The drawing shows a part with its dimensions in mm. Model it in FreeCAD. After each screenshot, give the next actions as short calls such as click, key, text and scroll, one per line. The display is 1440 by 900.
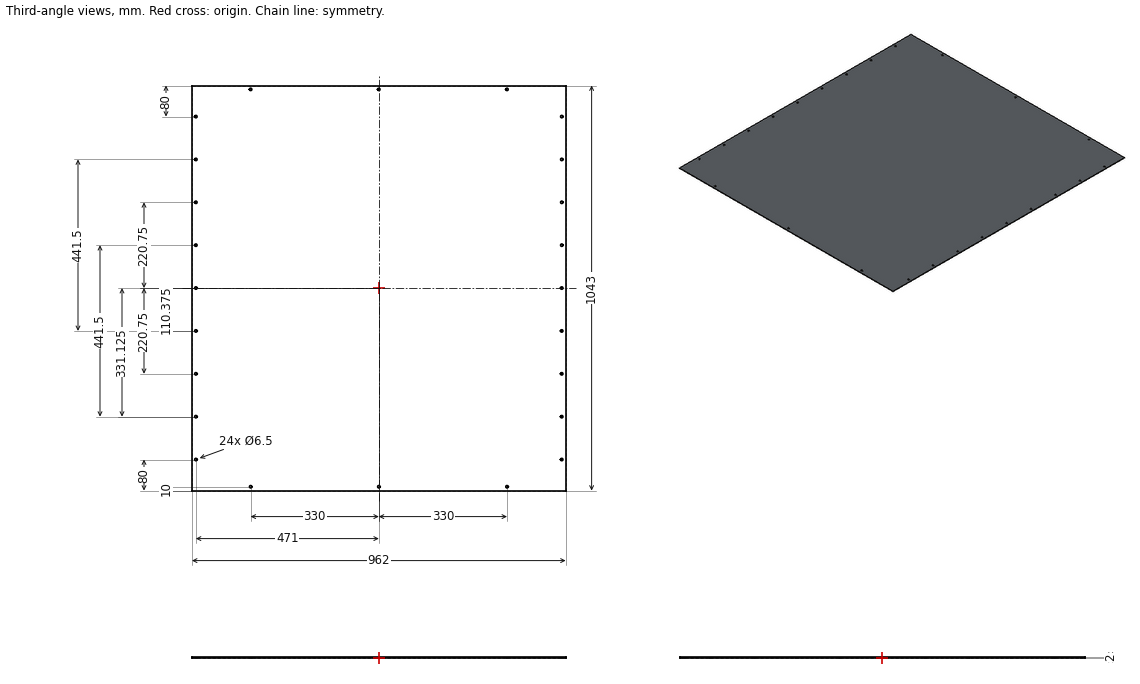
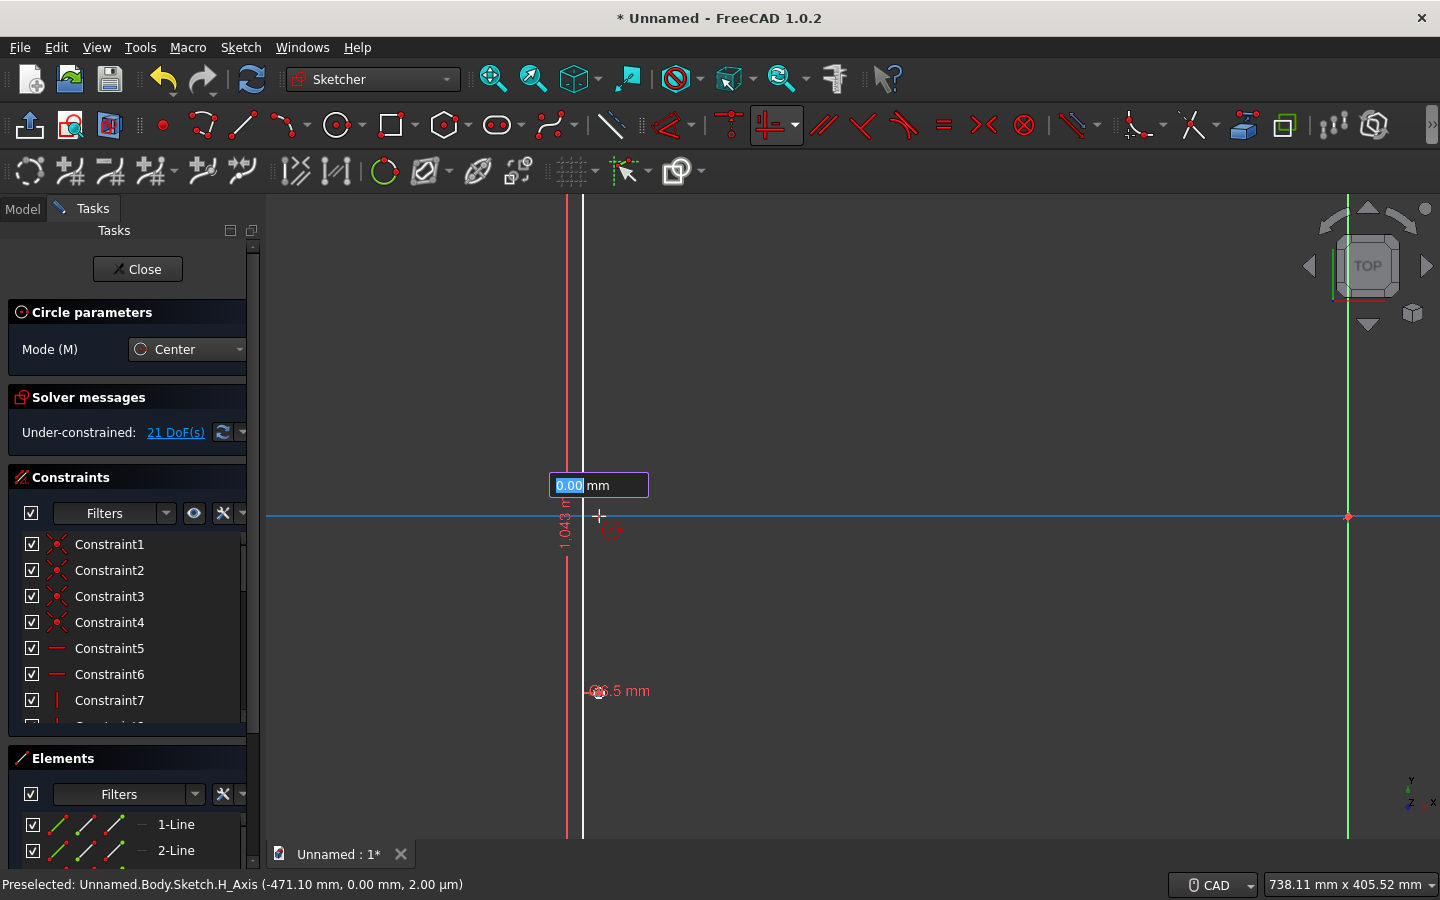
scroll(597, 521, up, 6)
move(598, 521)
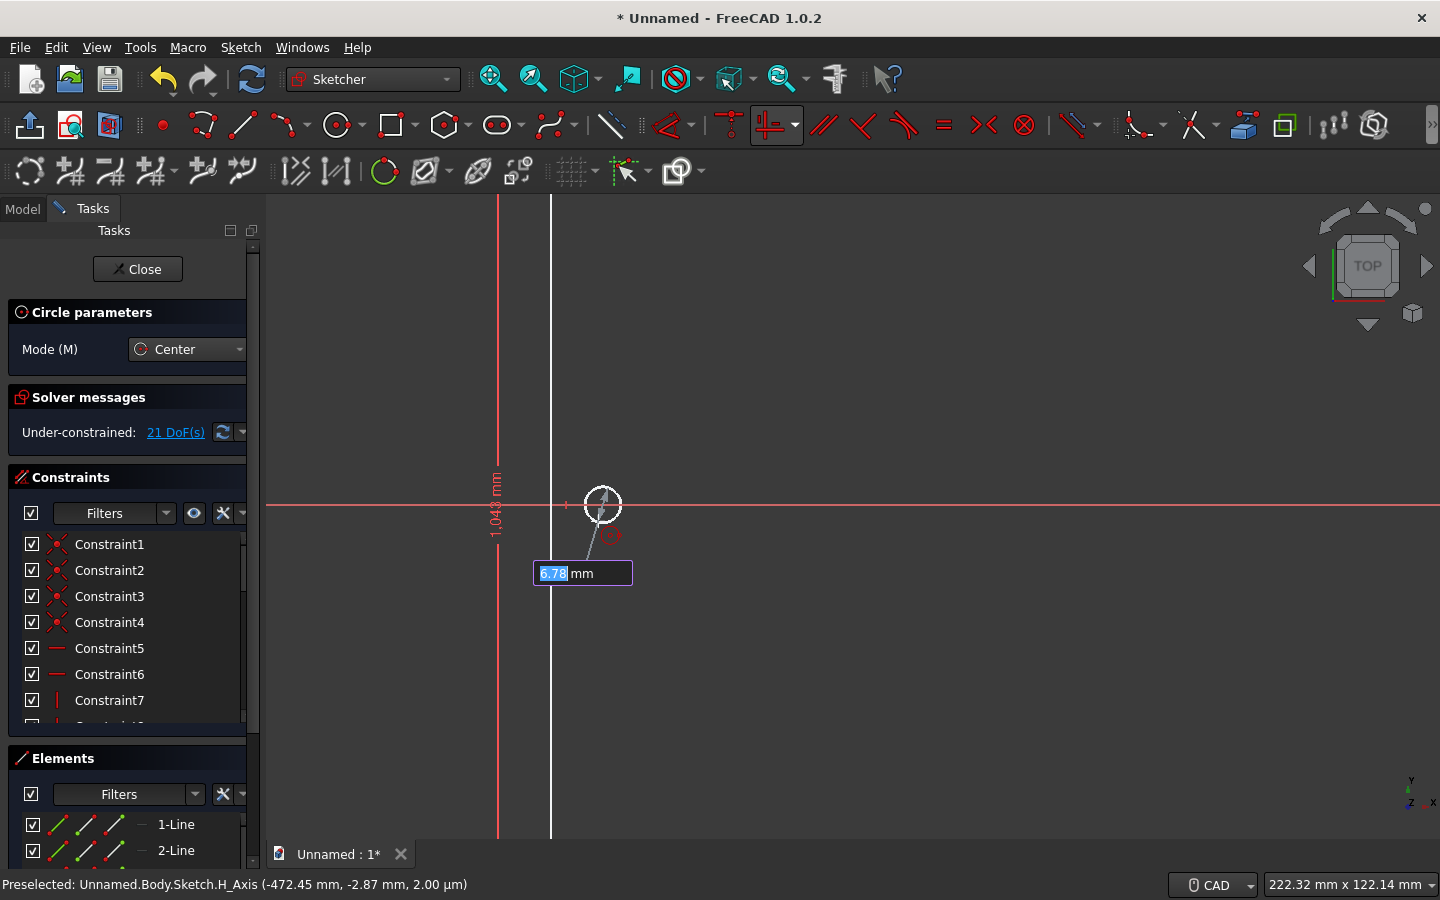
text(6.5)
key(Return)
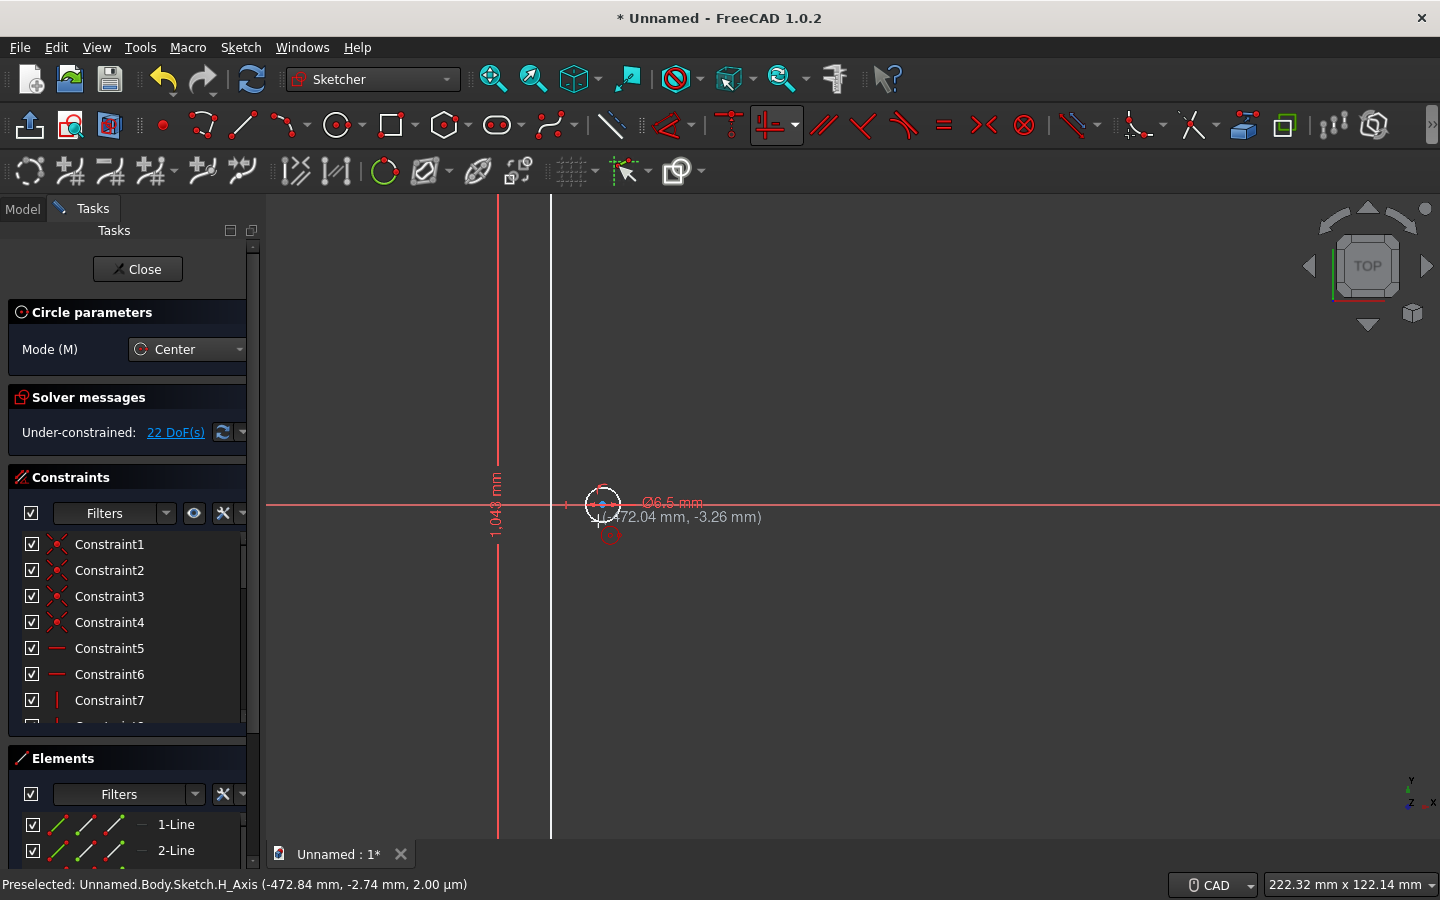
scroll(599, 517, down, 13)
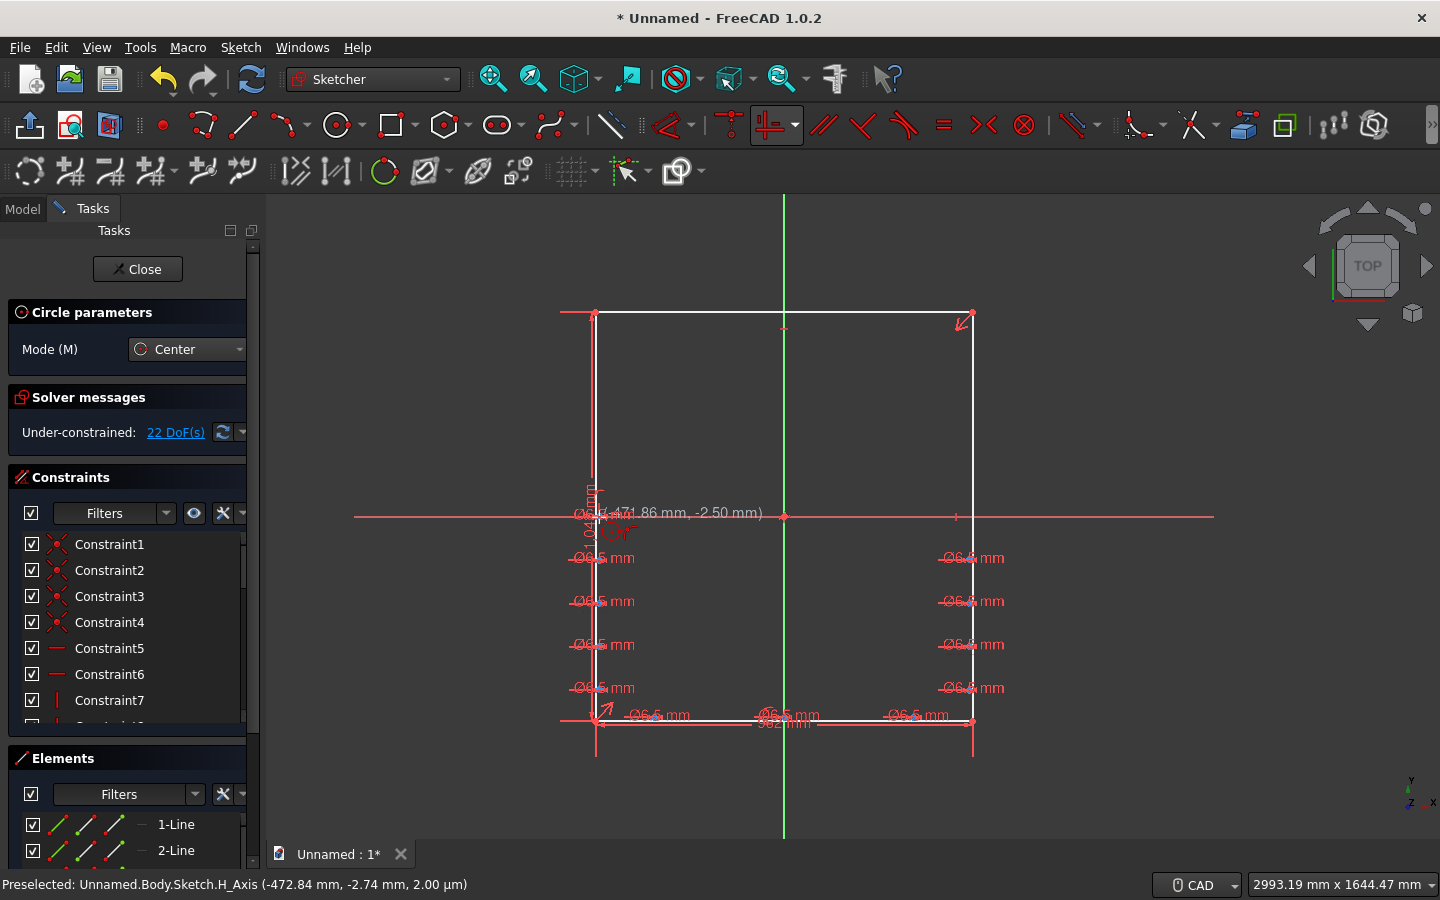
scroll(600, 473, up, 15)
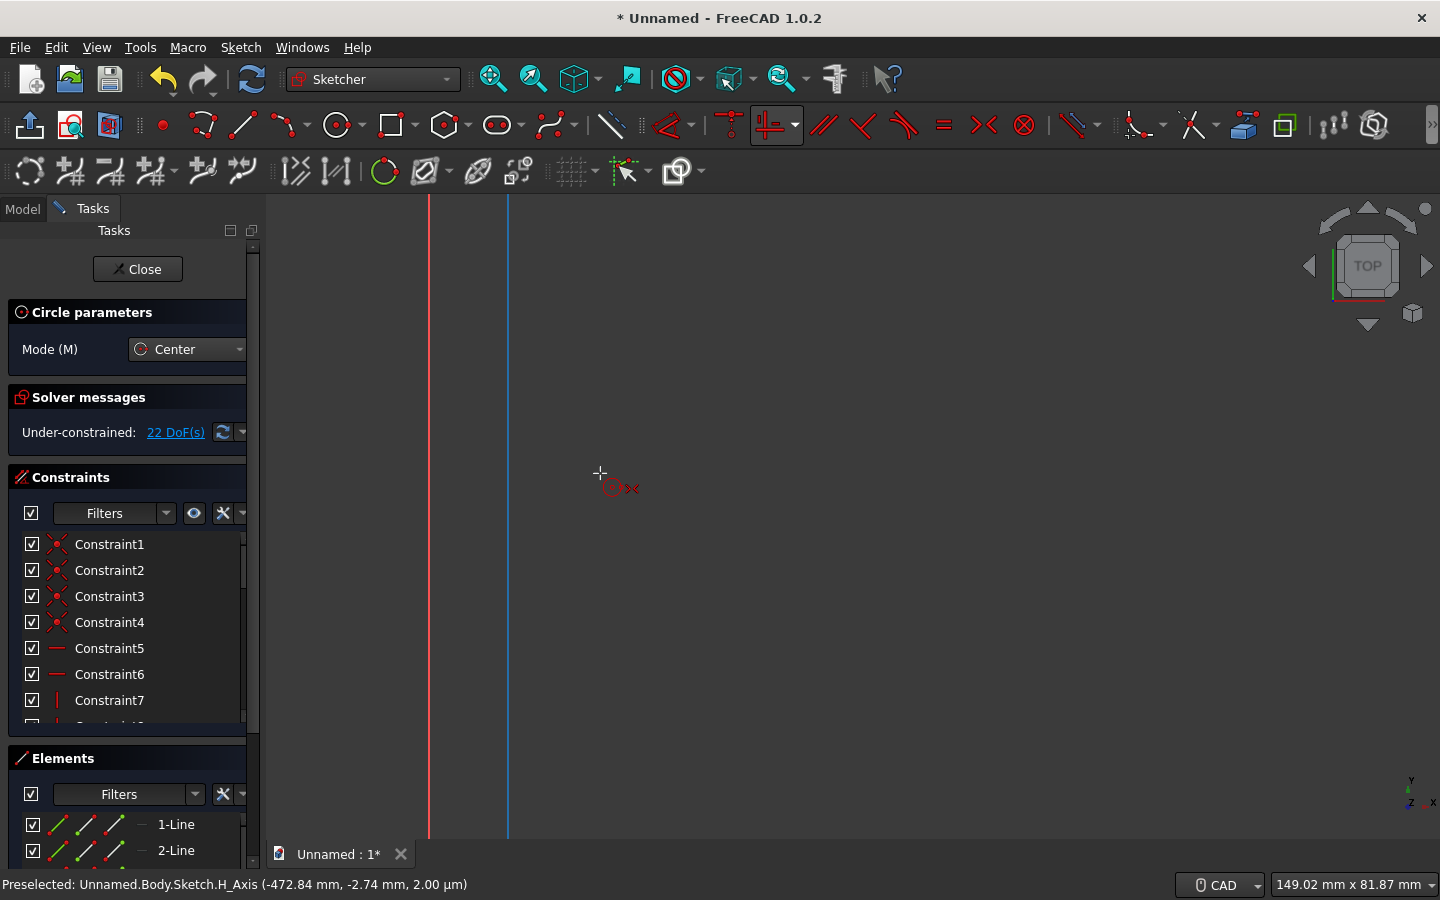
scroll(600, 473, down, 15)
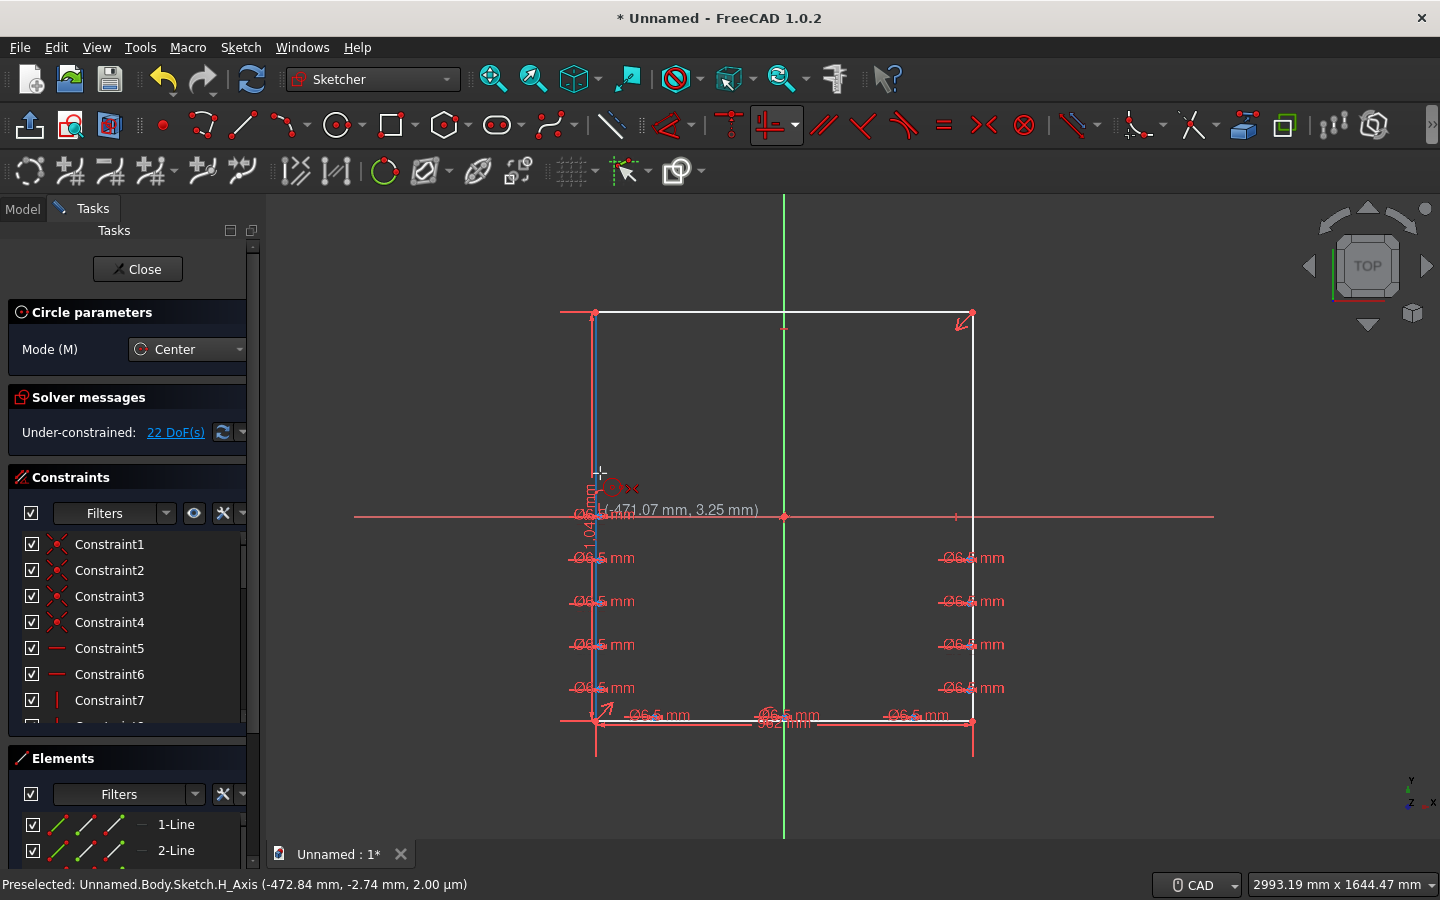
scroll(600, 473, up, 7)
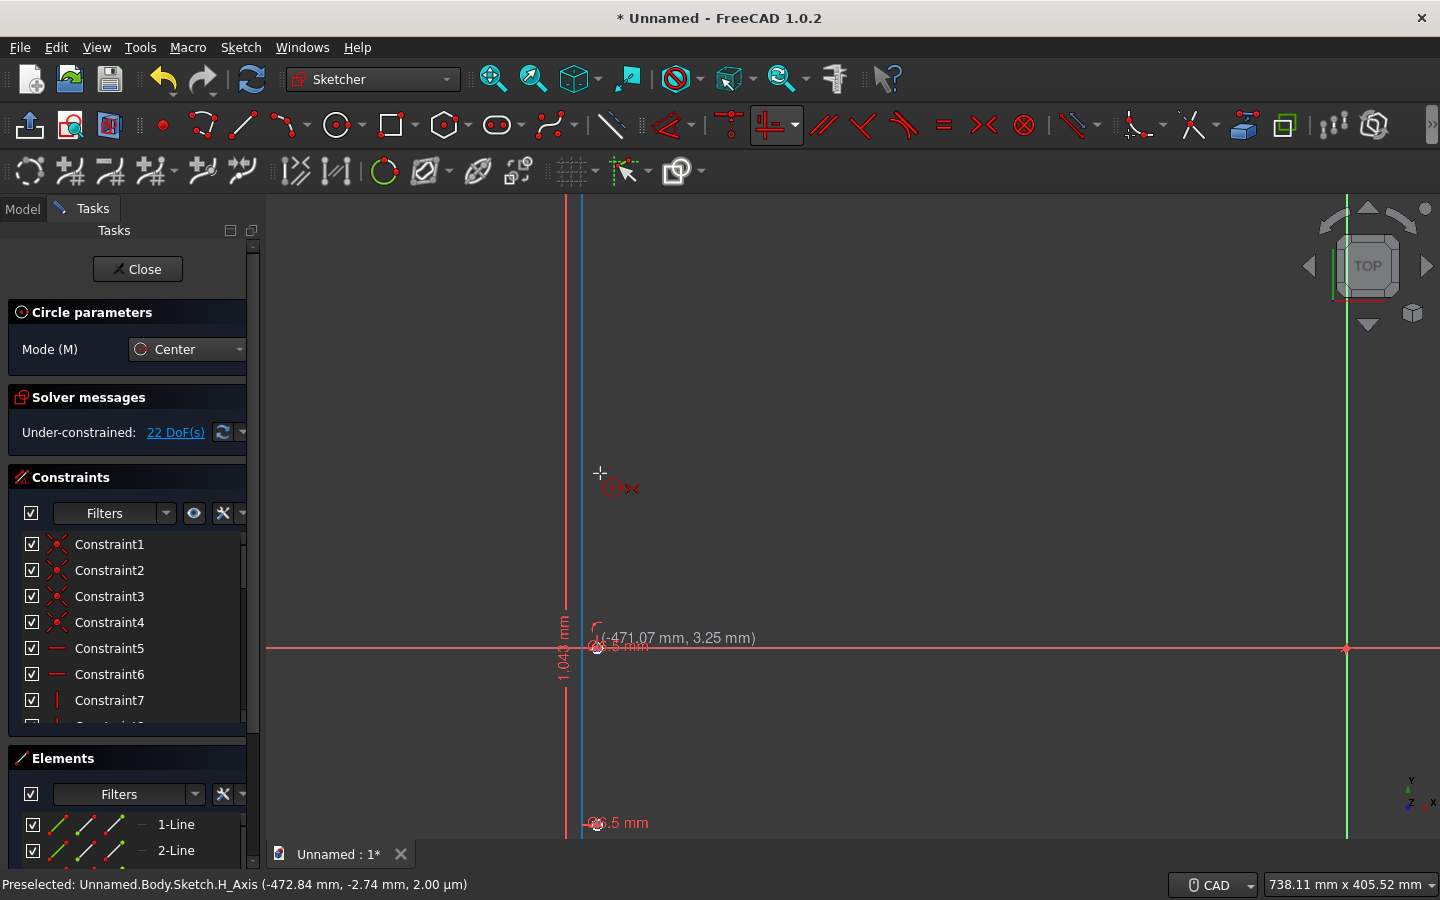
click(598, 473)
move(601, 469)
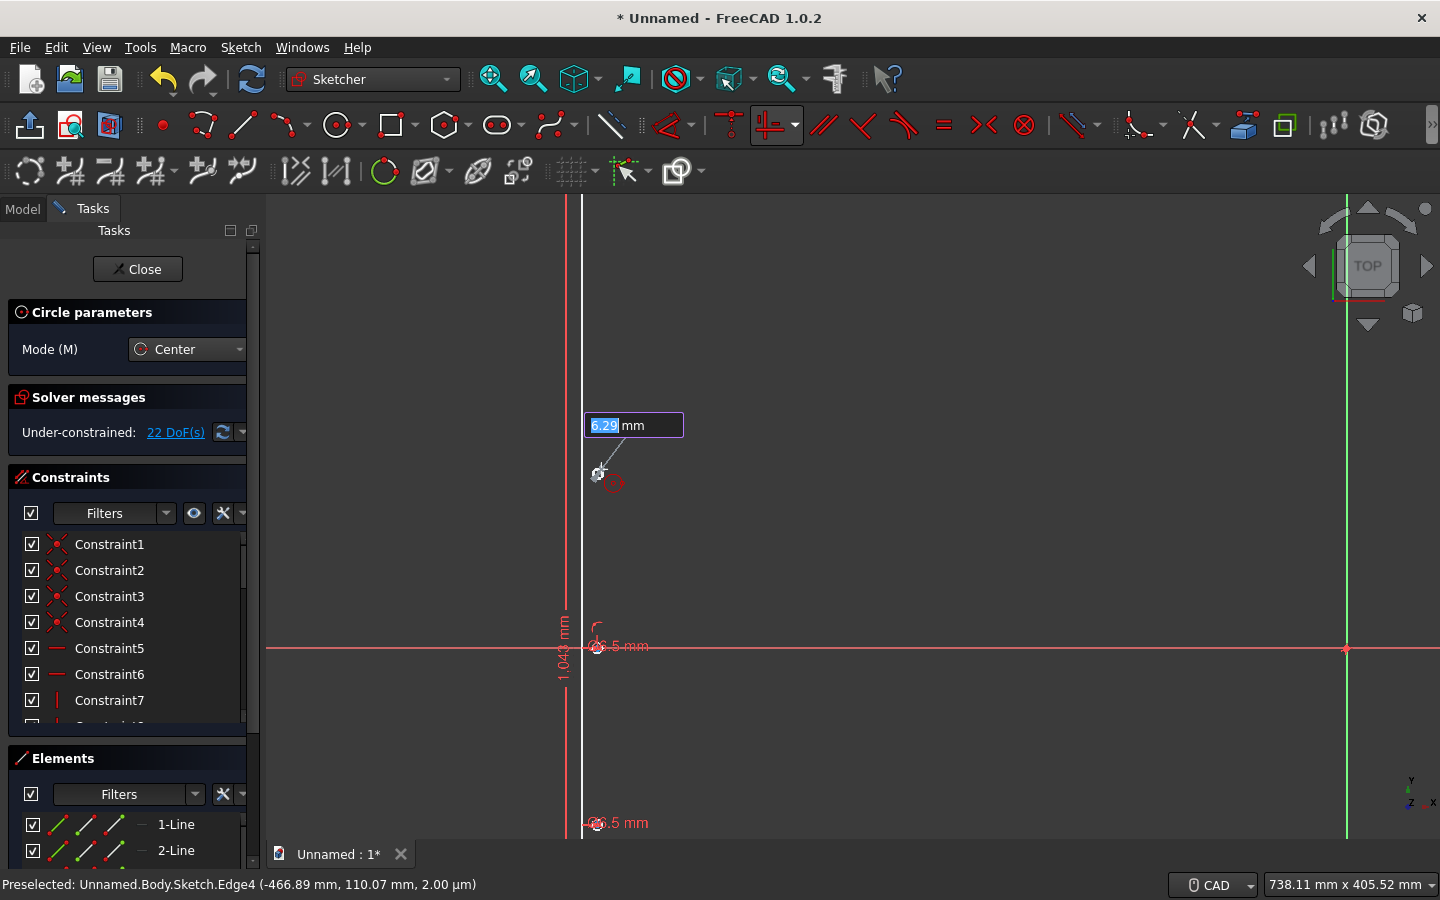
text(6.5)
key(Return)